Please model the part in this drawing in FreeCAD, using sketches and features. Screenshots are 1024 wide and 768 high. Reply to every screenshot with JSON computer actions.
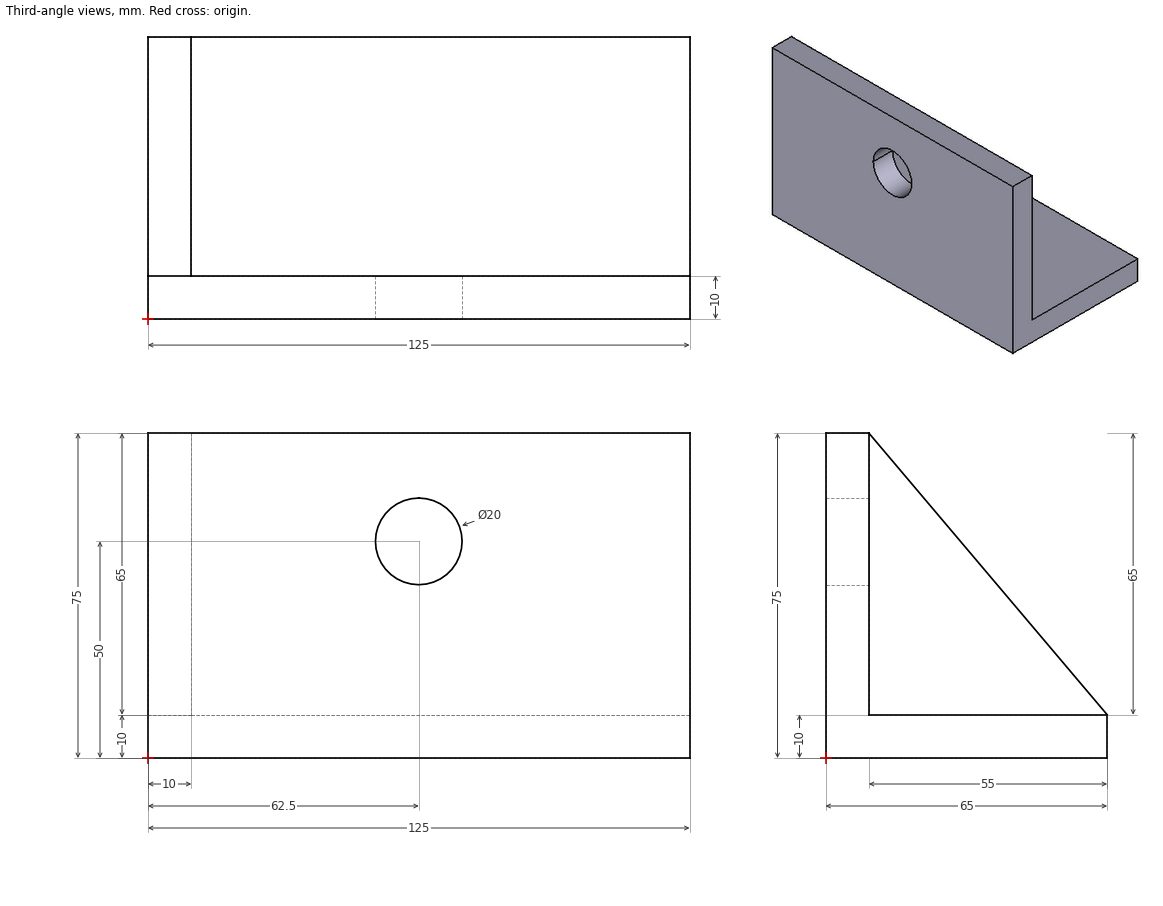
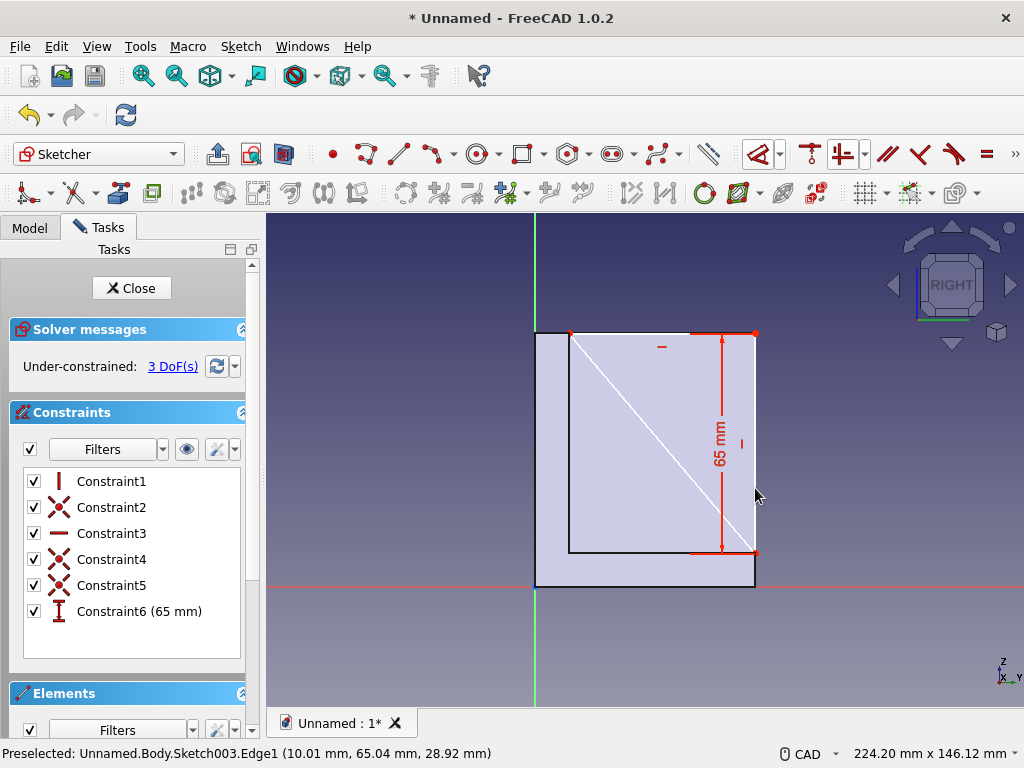
{"action": "left_click", "coordinate": [699, 334]}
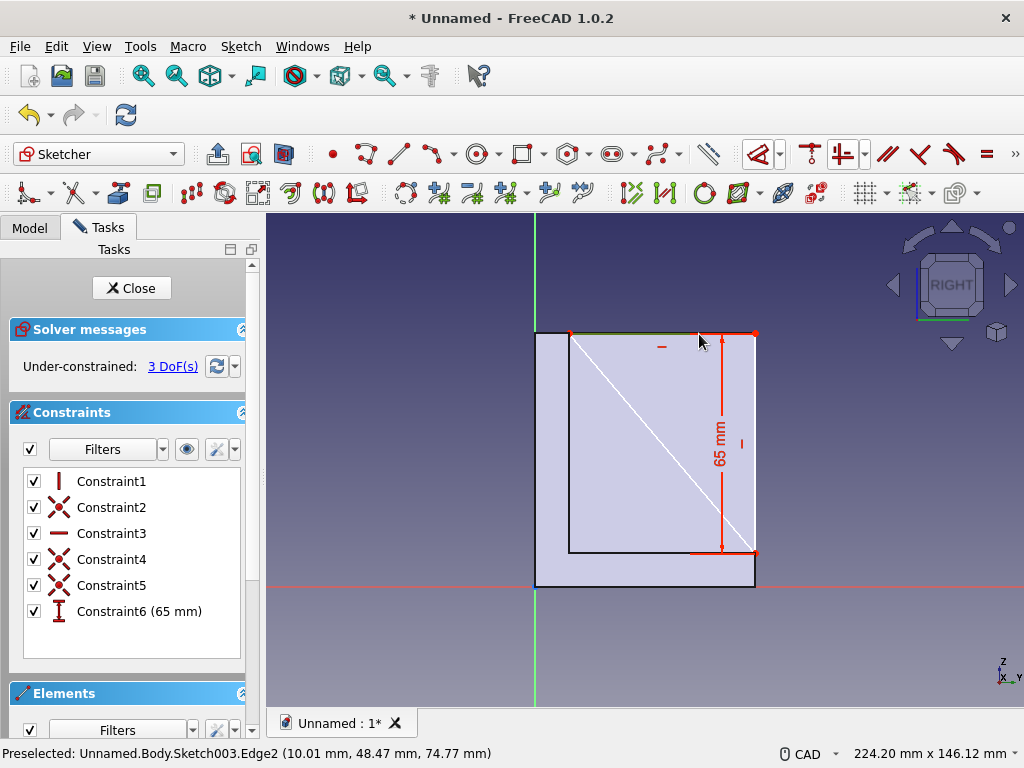
{"action": "key", "text": "l"}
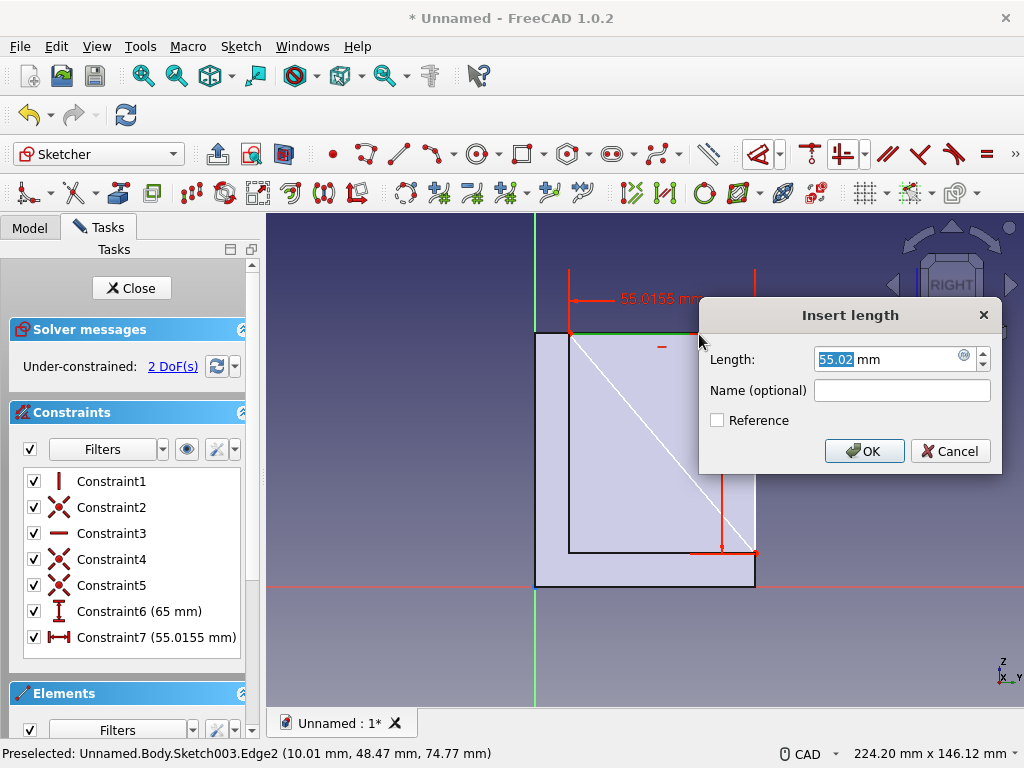
{"action": "type", "text": "55"}
{"action": "key", "text": "Return"}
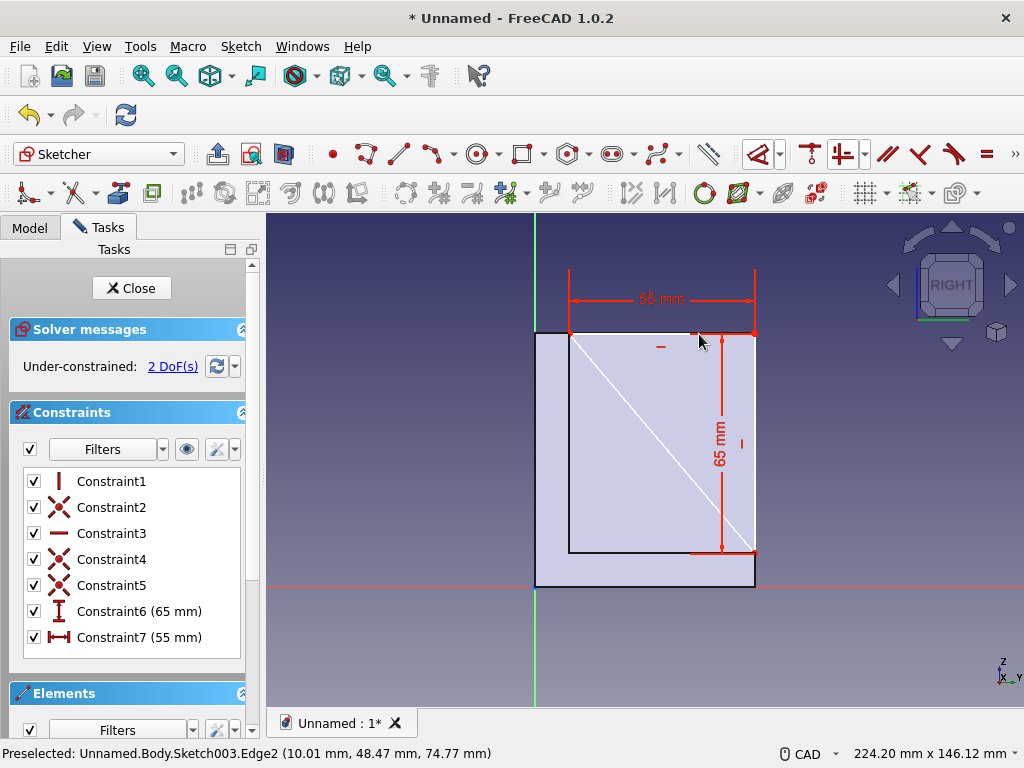
{"action": "left_click", "coordinate": [755, 554]}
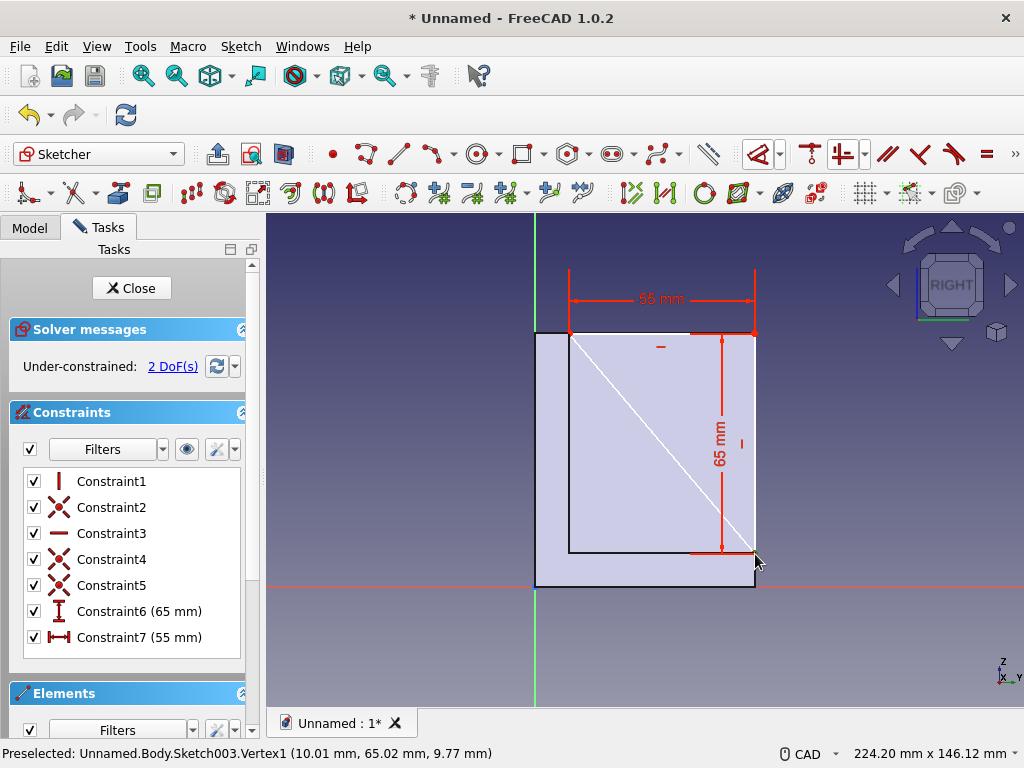
{"action": "key", "text": "l"}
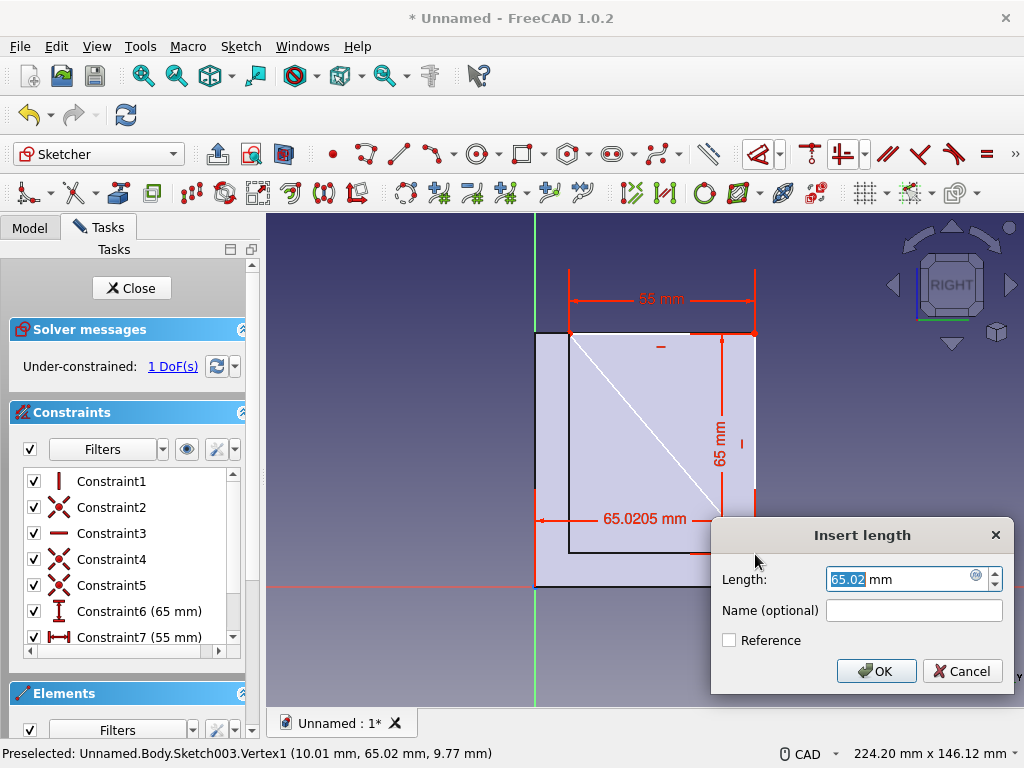
{"action": "type", "text": "65"}
{"action": "key", "text": "Return"}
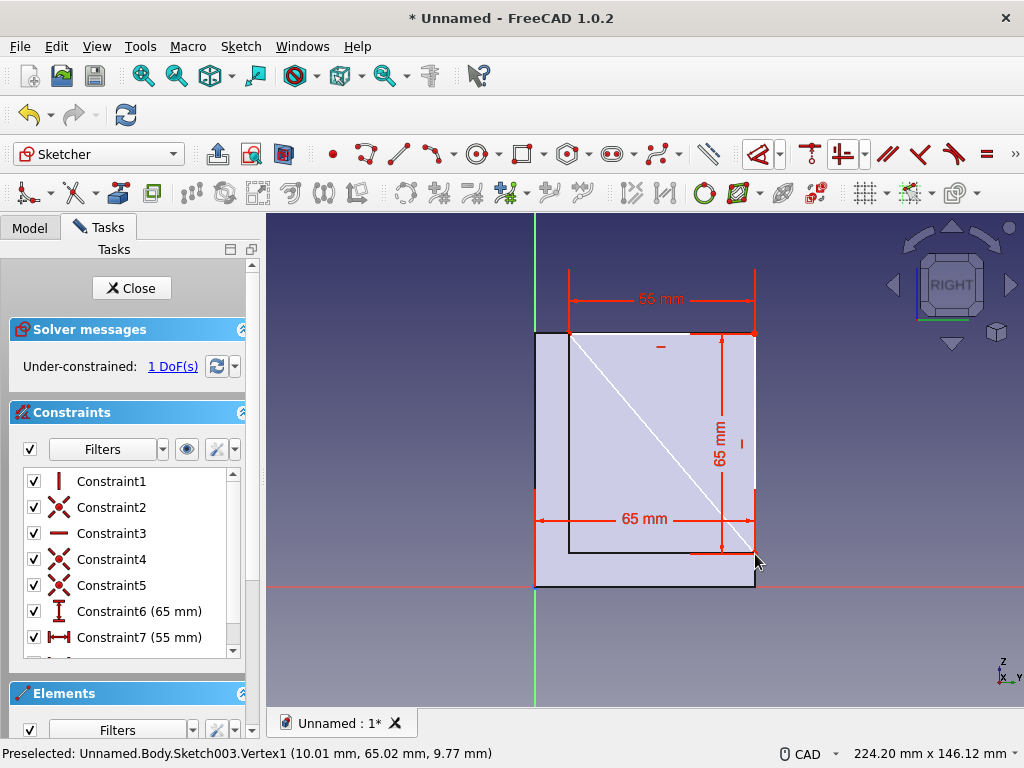
{"action": "left_click", "coordinate": [755, 554]}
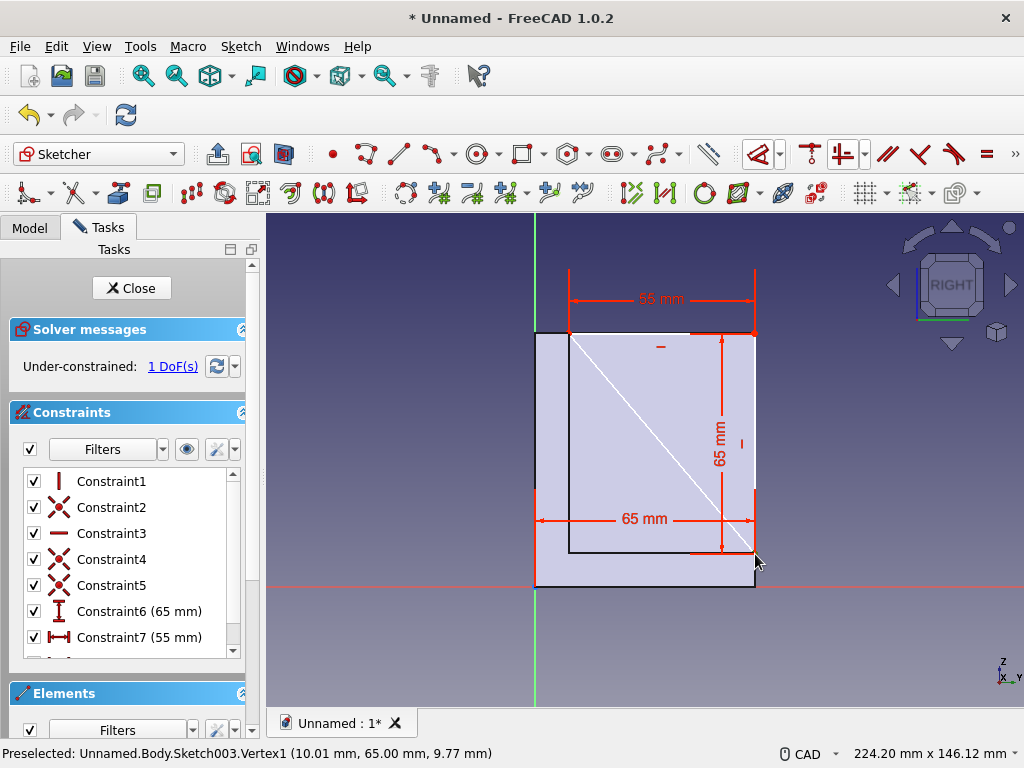
{"action": "key", "text": "i"}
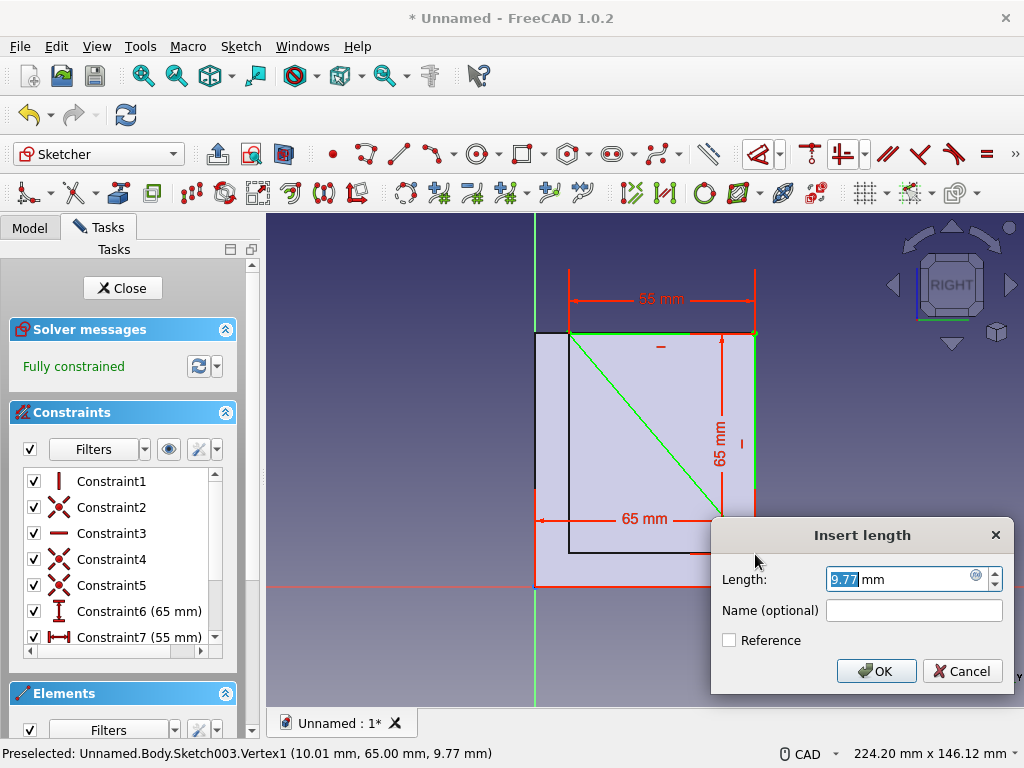
{"action": "type", "text": "10"}
{"action": "key", "text": "Return"}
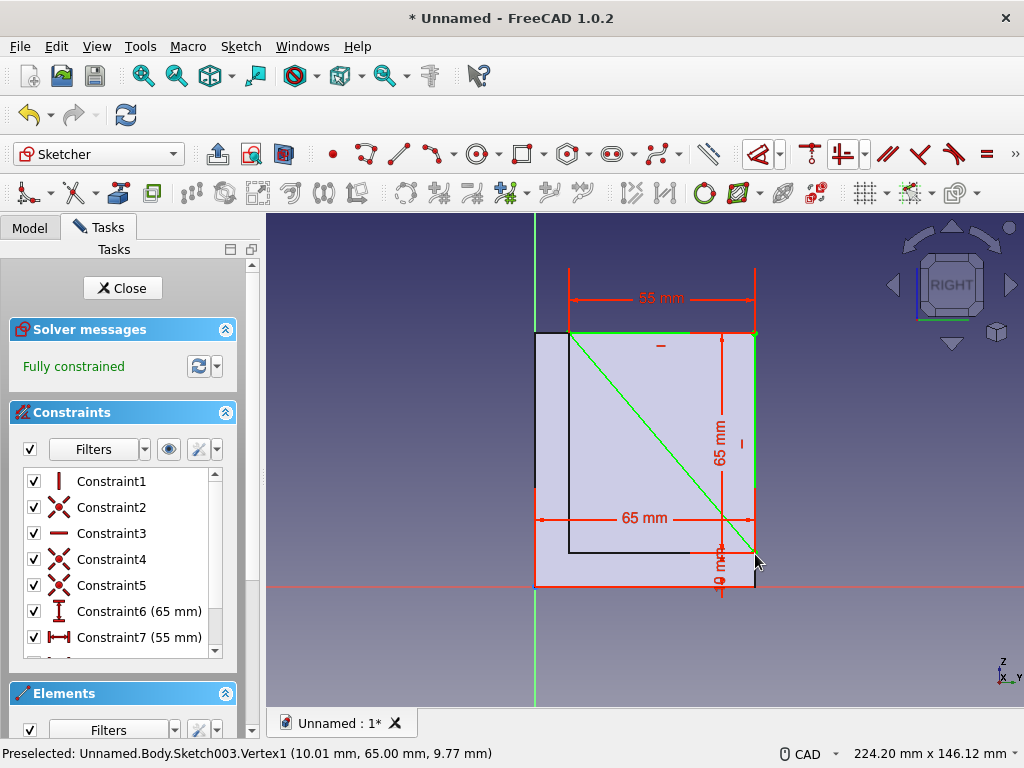
{"action": "left_click", "coordinate": [123, 288]}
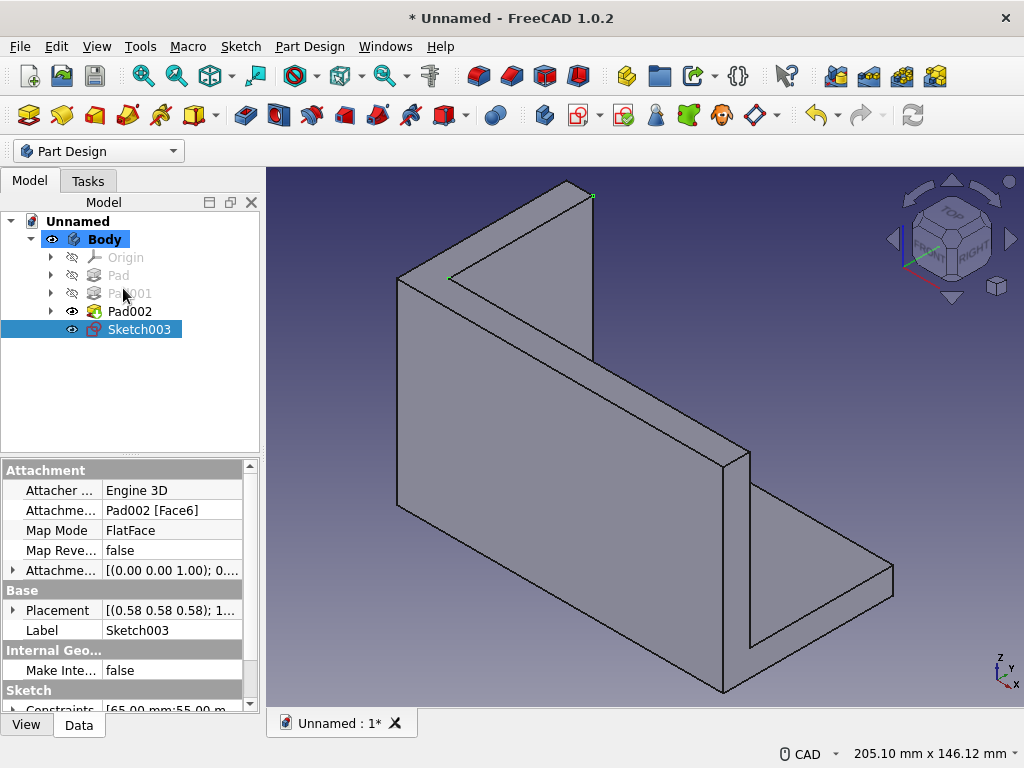
{"action": "left_click", "coordinate": [246, 116]}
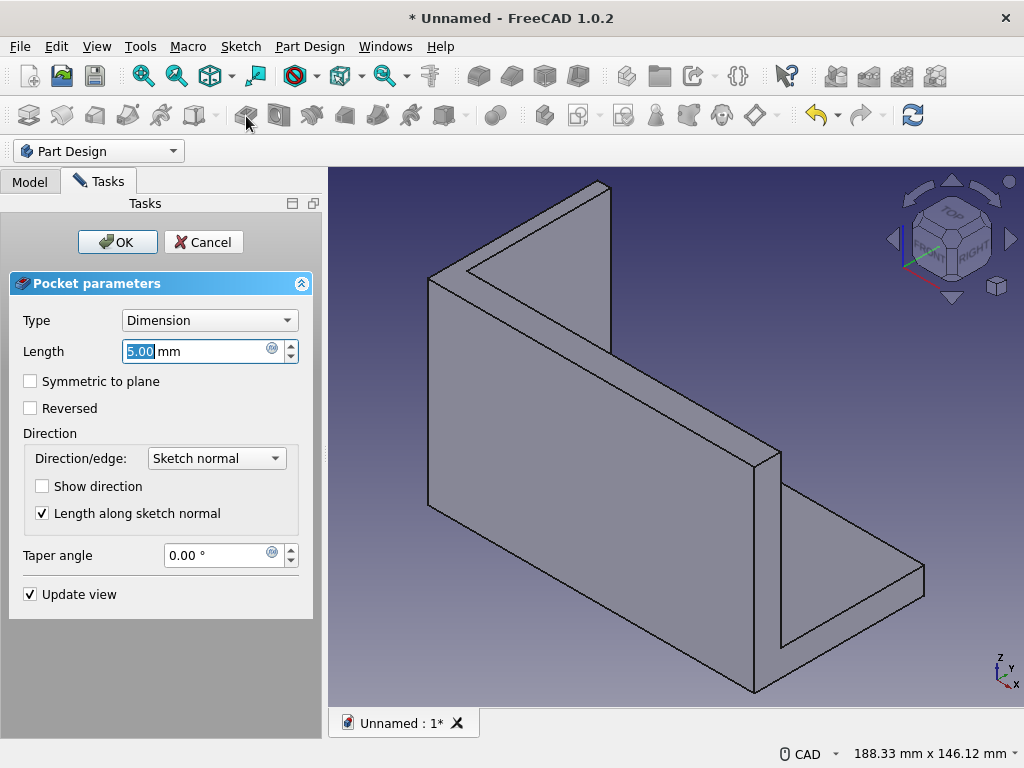
{"action": "type", "text": "55"}
{"action": "key", "text": "Tab"}